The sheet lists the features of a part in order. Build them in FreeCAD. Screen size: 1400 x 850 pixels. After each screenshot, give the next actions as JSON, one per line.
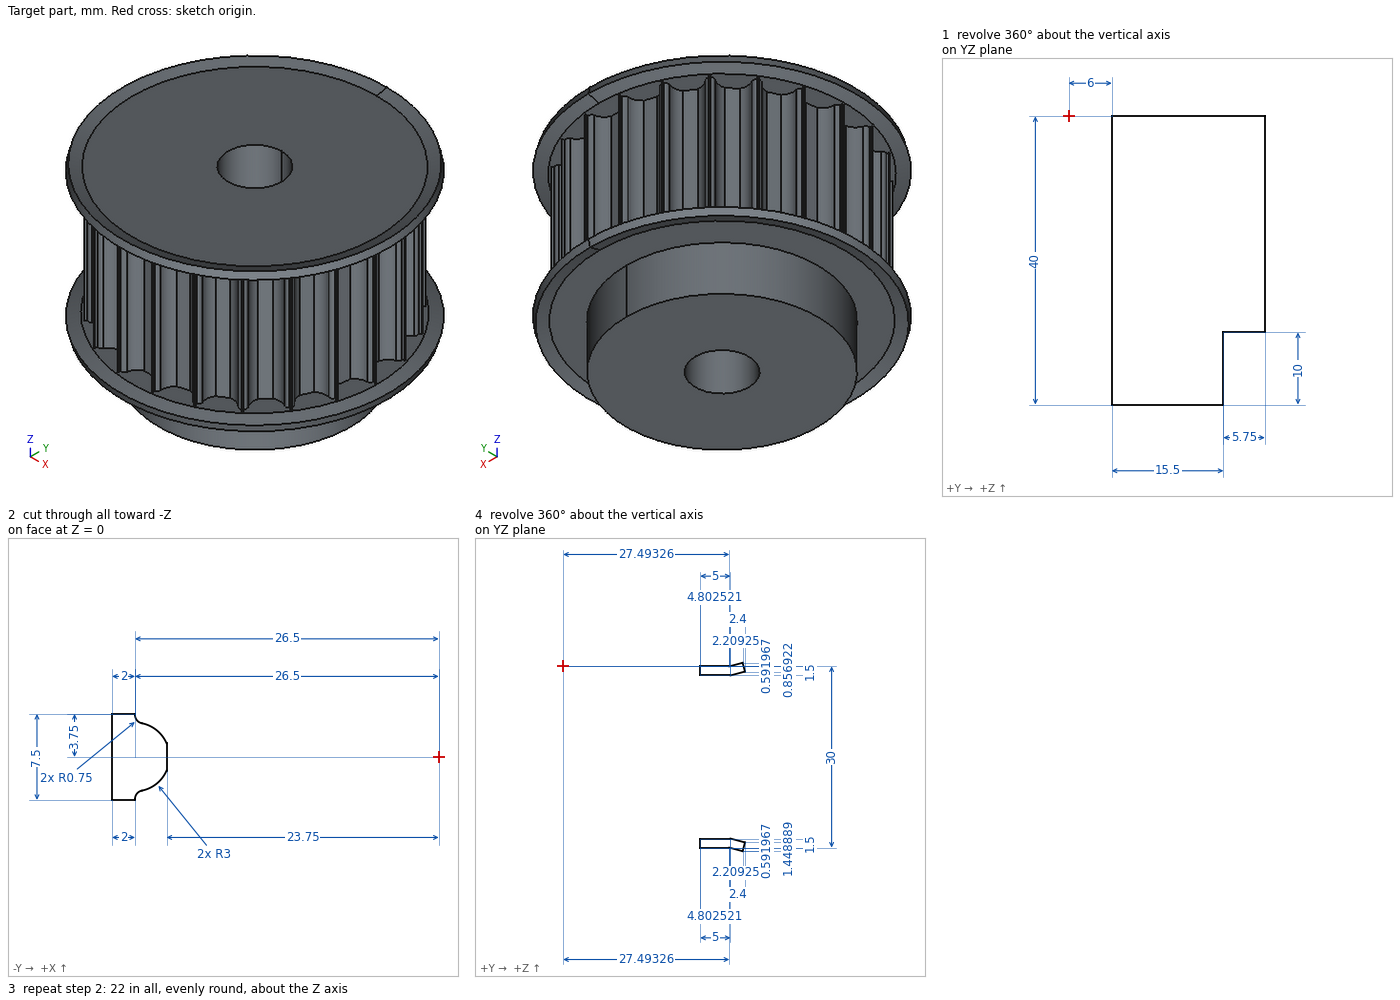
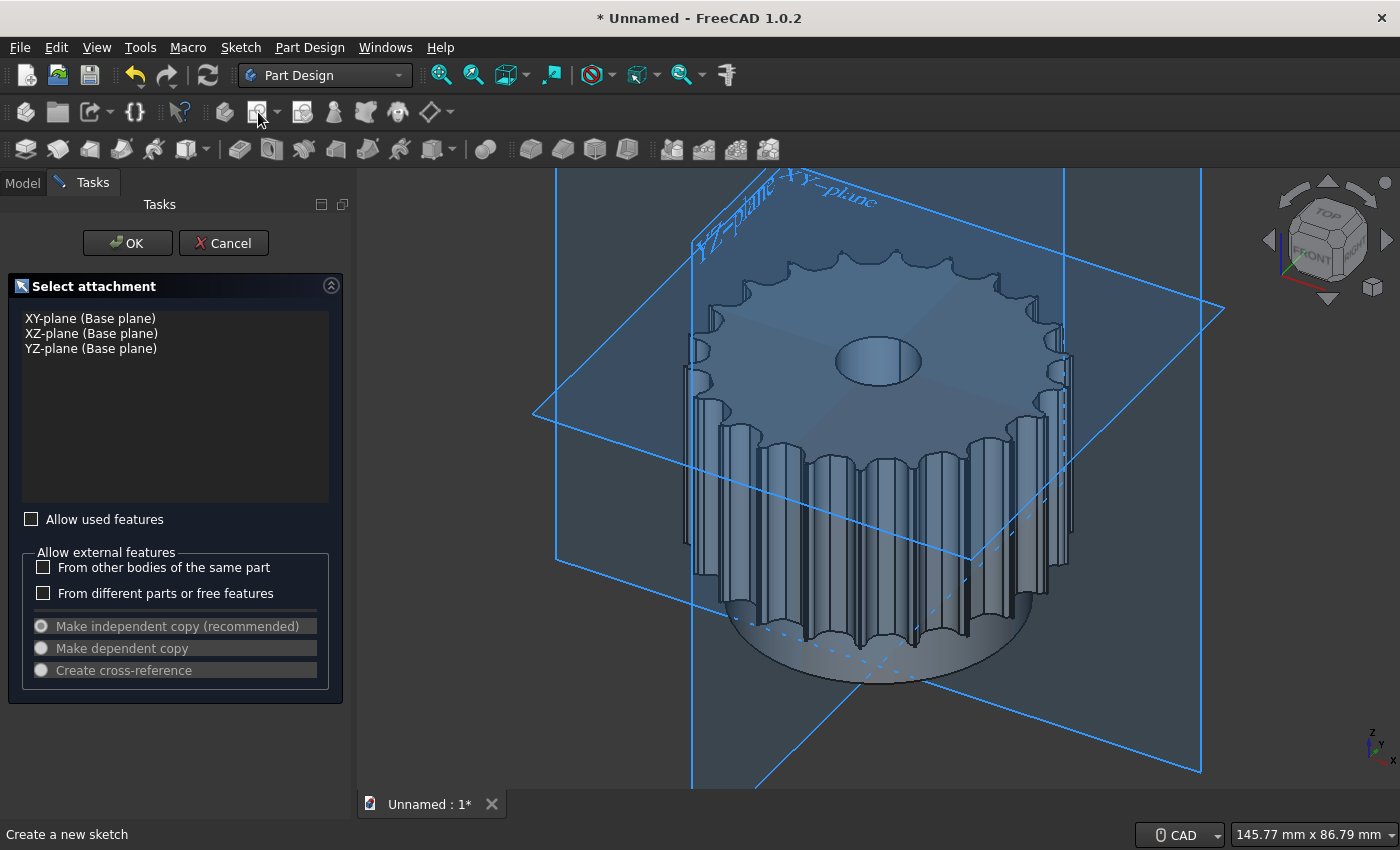
{"action": "left_click", "coordinate": [82, 348]}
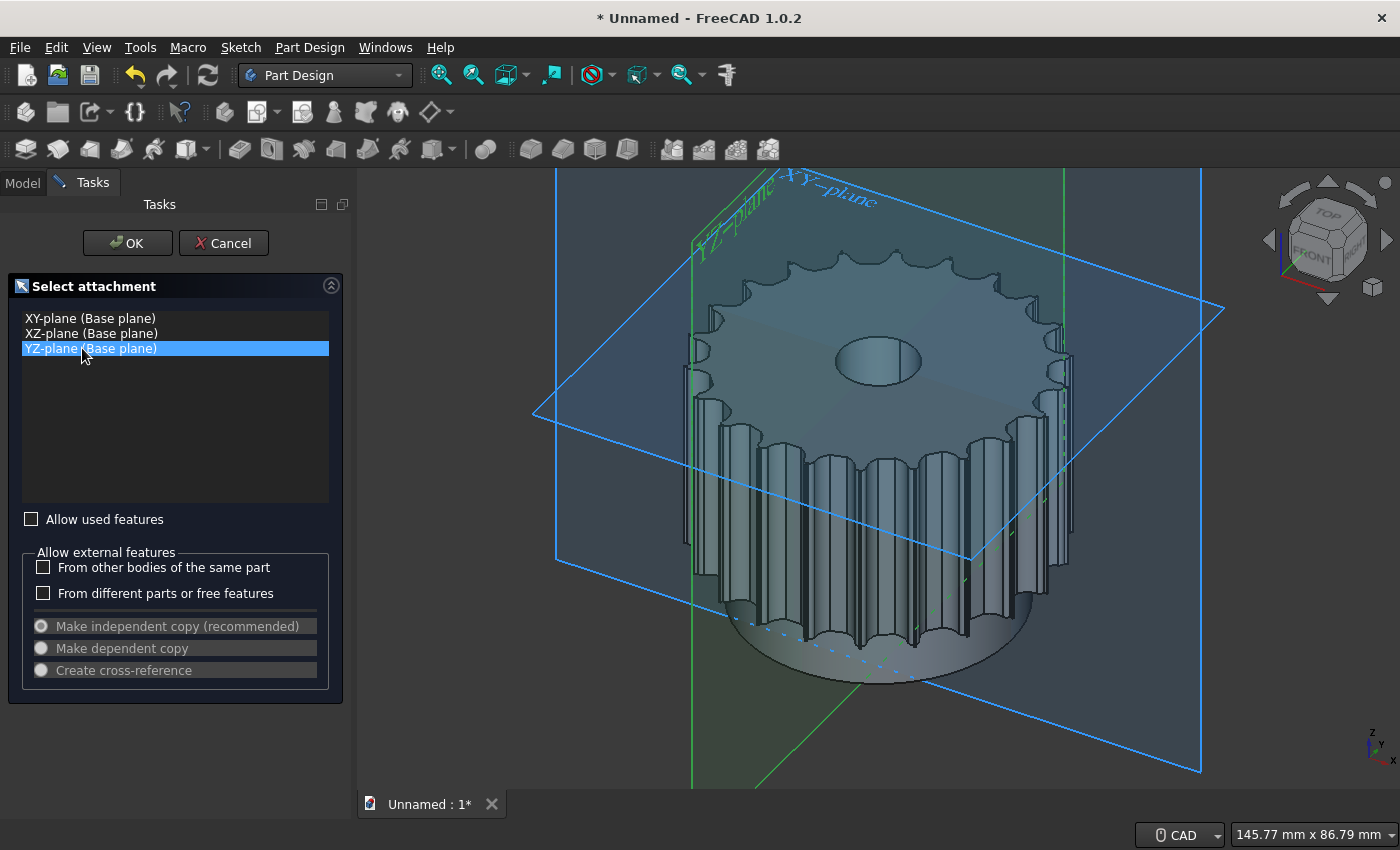
{"action": "left_click", "coordinate": [128, 243]}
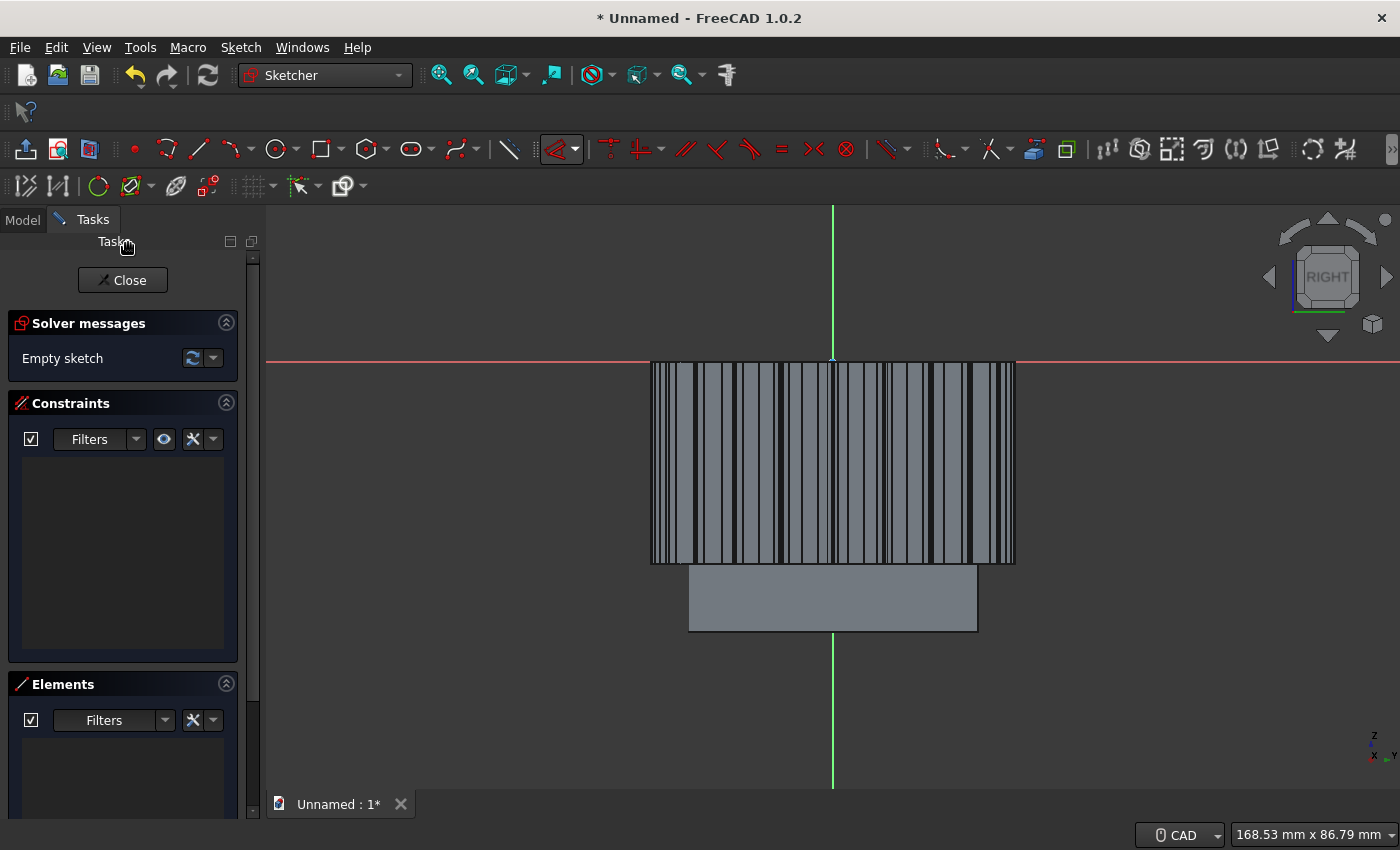
{"action": "key", "text": "q s"}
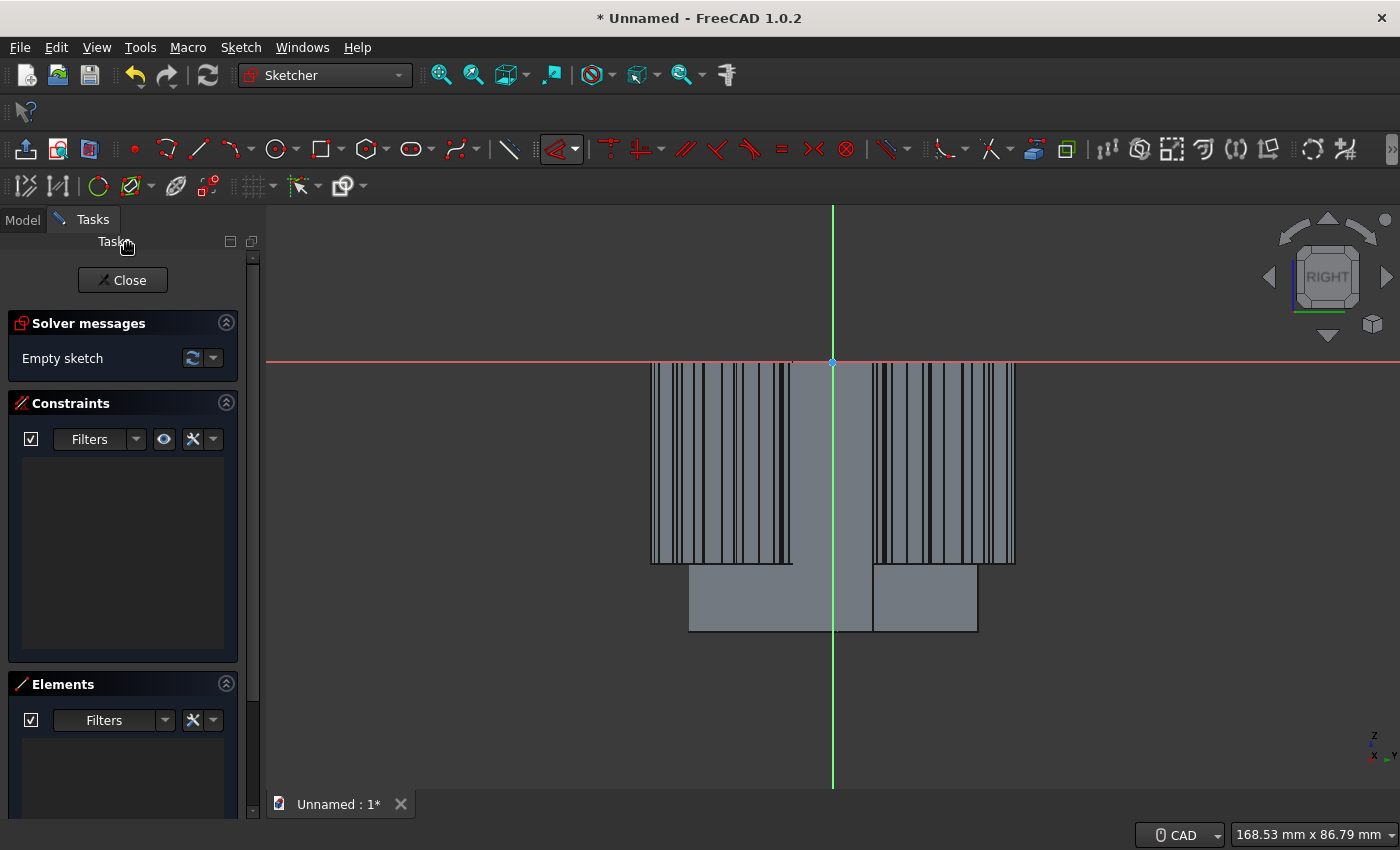
{"action": "scroll", "coordinate": [1141, 423], "scroll_direction": "up", "scroll_amount": 3}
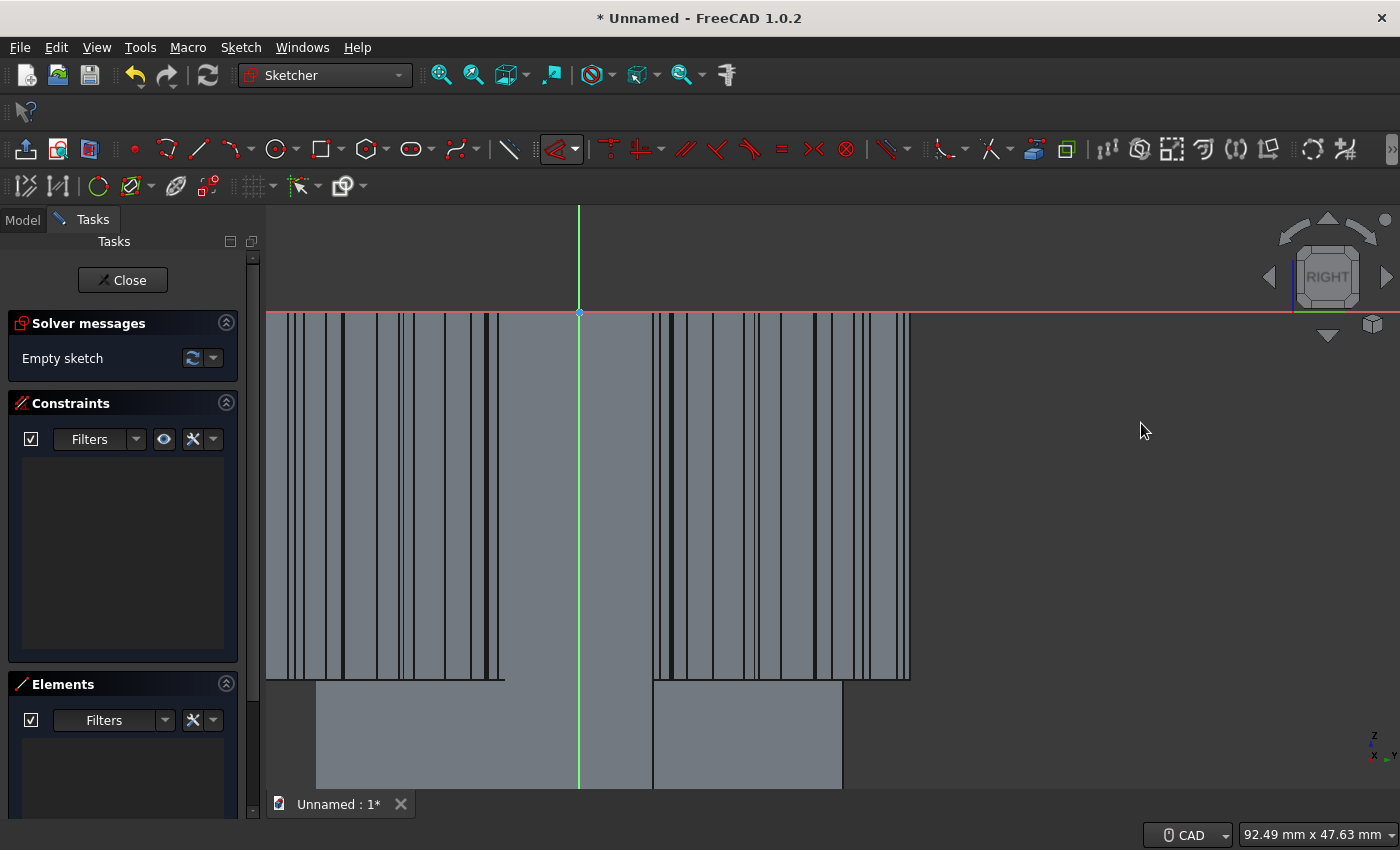
{"action": "left_click", "coordinate": [168, 150]}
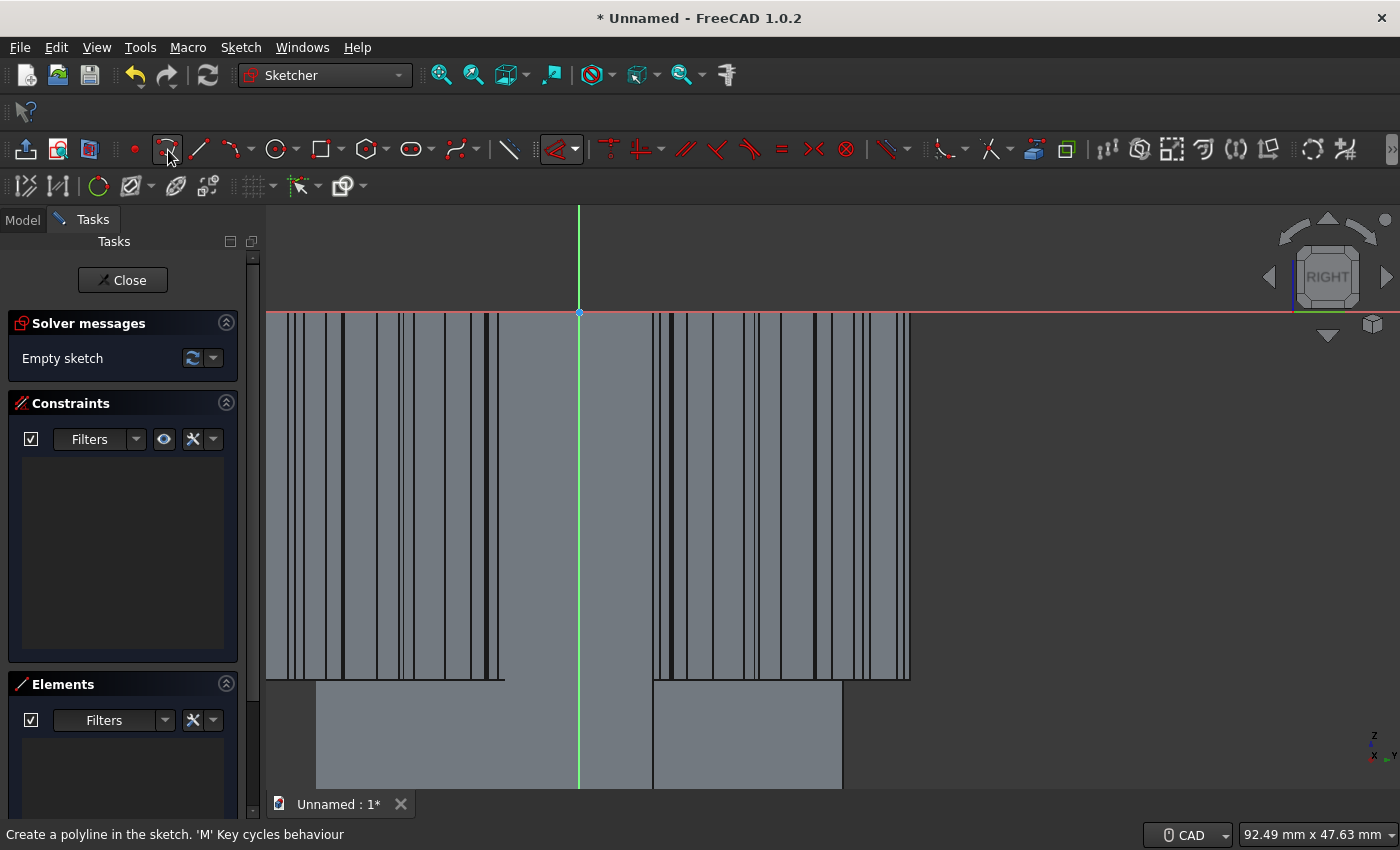
{"action": "left_click", "coordinate": [857, 312]}
{"action": "left_click", "coordinate": [857, 331]}
{"action": "left_click", "coordinate": [919, 331]}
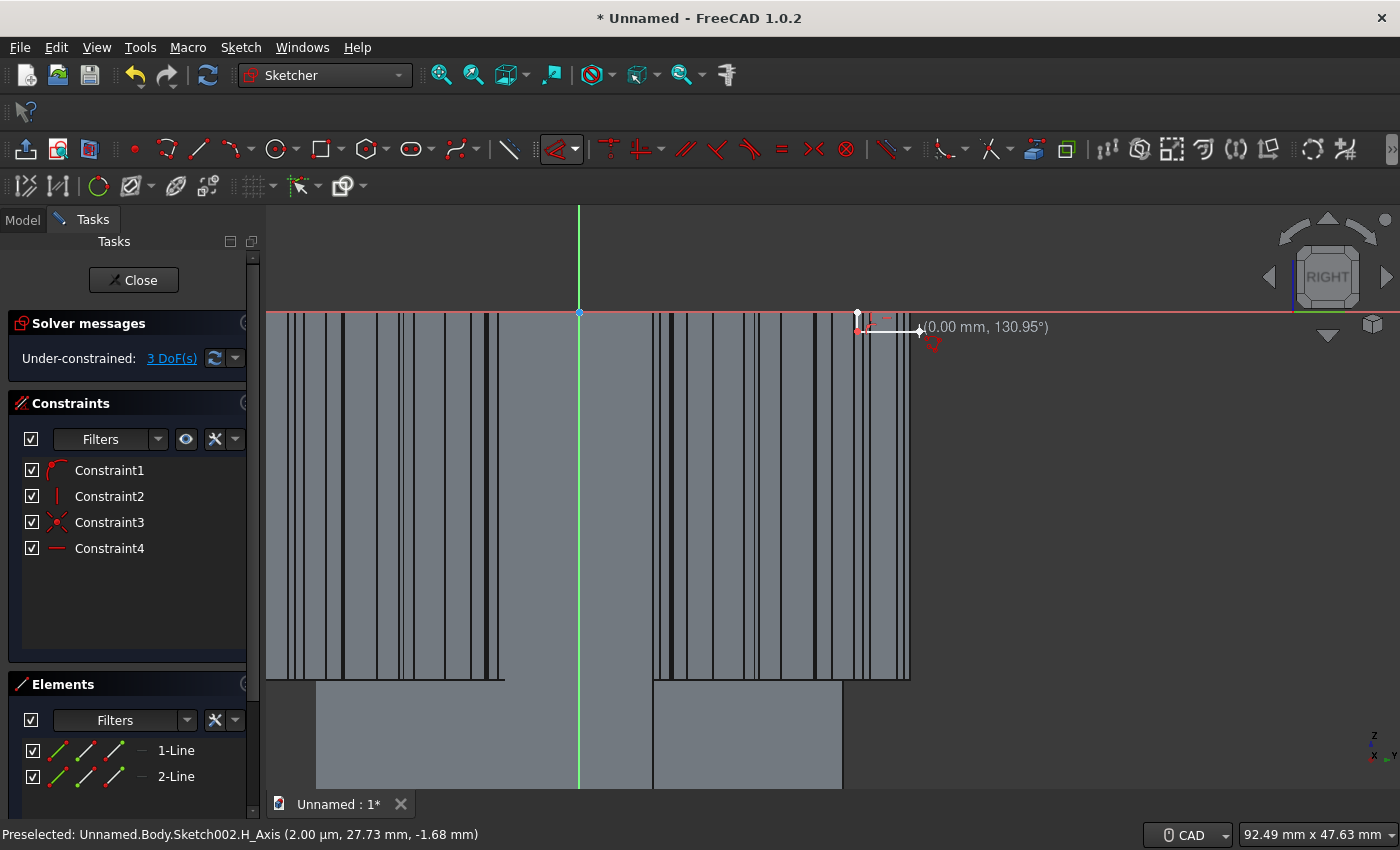
{"action": "scroll", "coordinate": [948, 323], "scroll_direction": "up", "scroll_amount": 3}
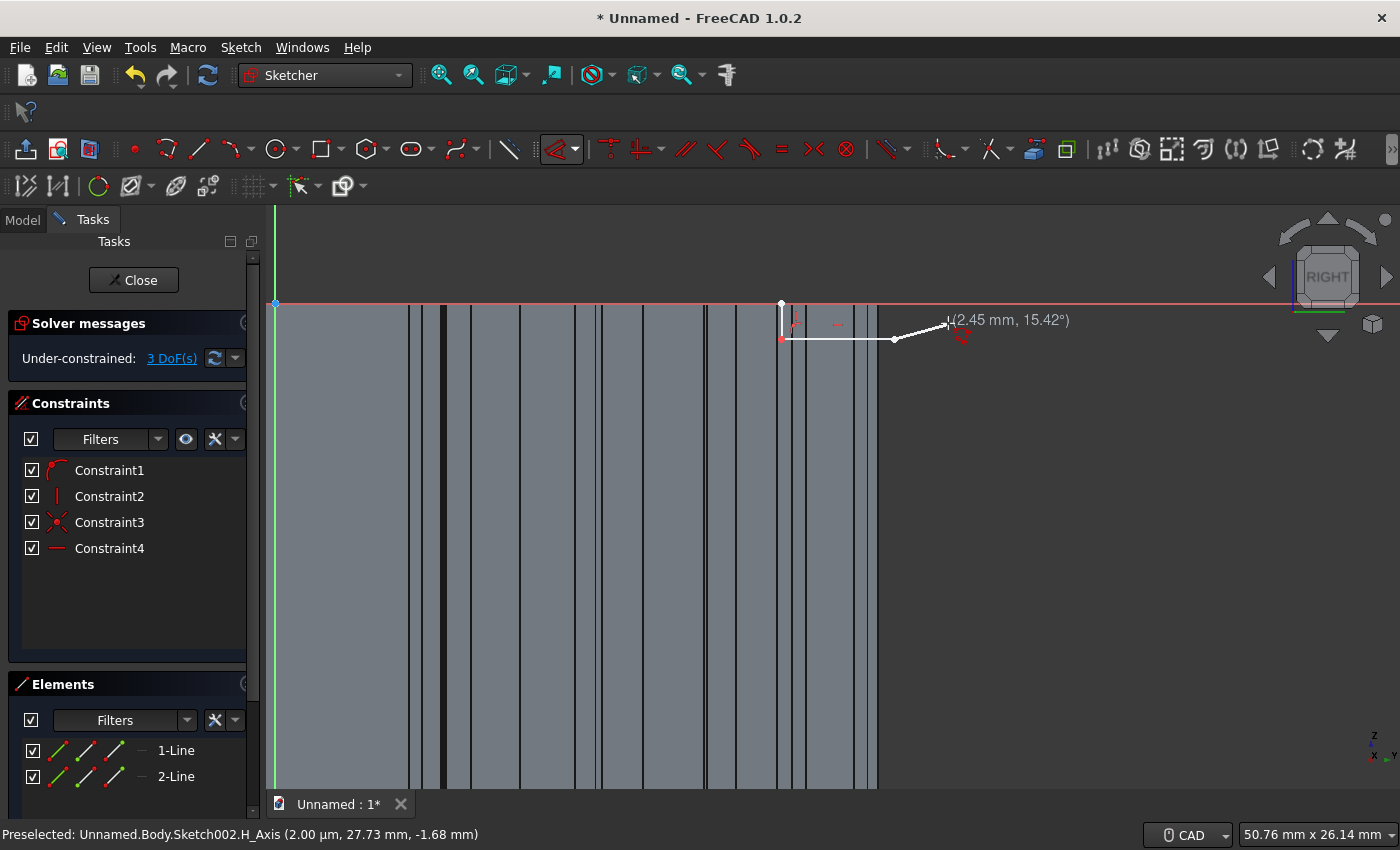
{"action": "left_click", "coordinate": [947, 323]}
{"action": "left_click", "coordinate": [939, 290]}
{"action": "left_click", "coordinate": [889, 313]}
{"action": "left_click", "coordinate": [782, 304]}